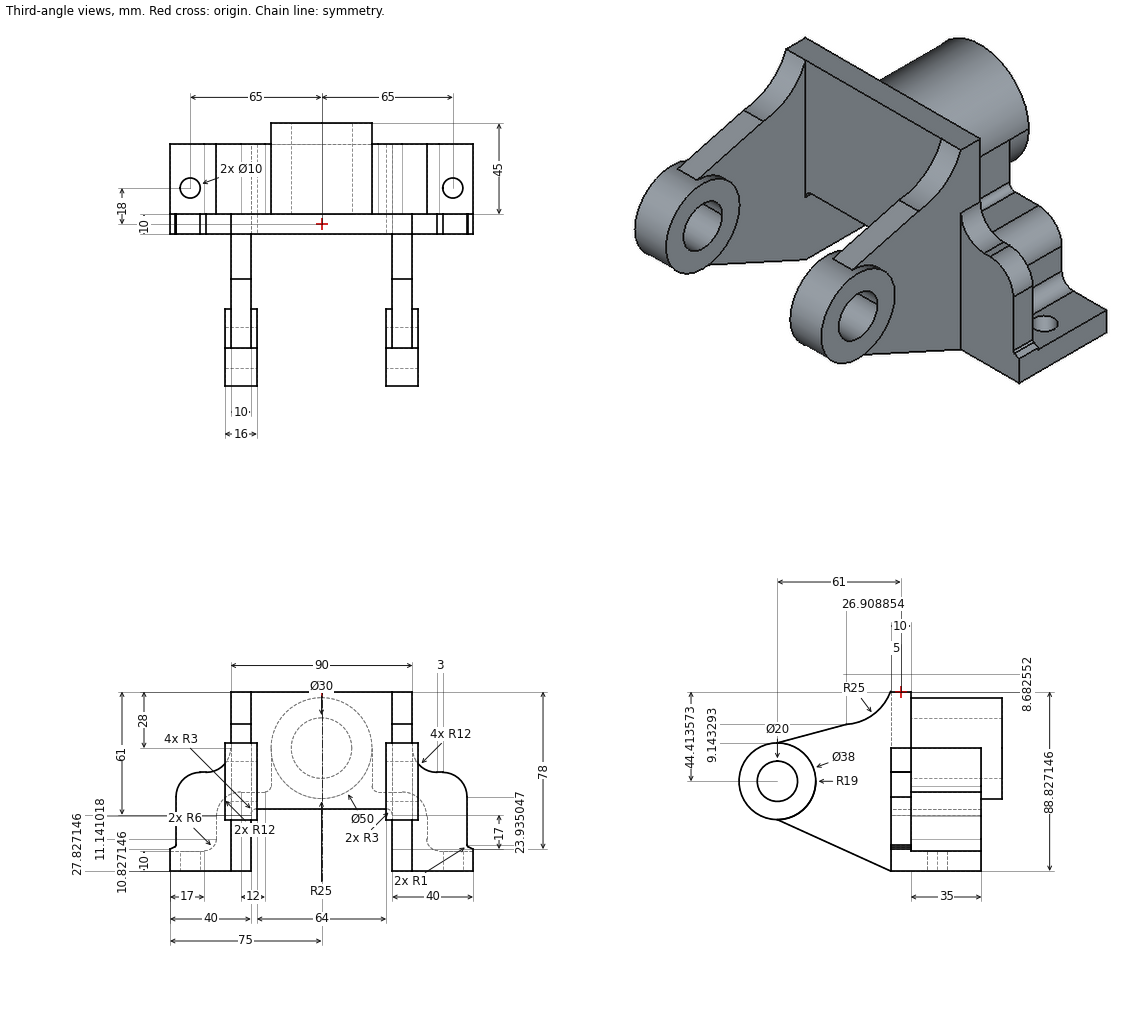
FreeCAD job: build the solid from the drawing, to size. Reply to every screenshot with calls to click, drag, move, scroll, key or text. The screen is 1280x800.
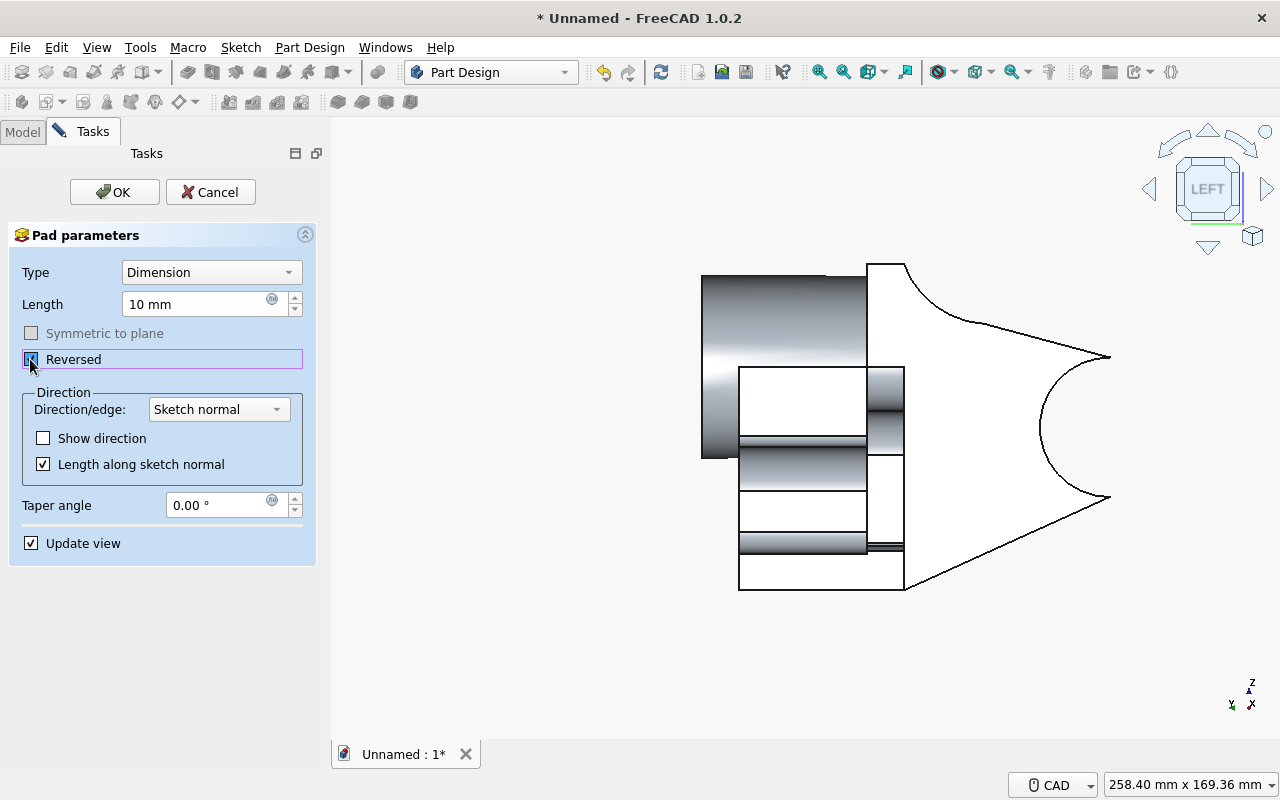
click(115, 192)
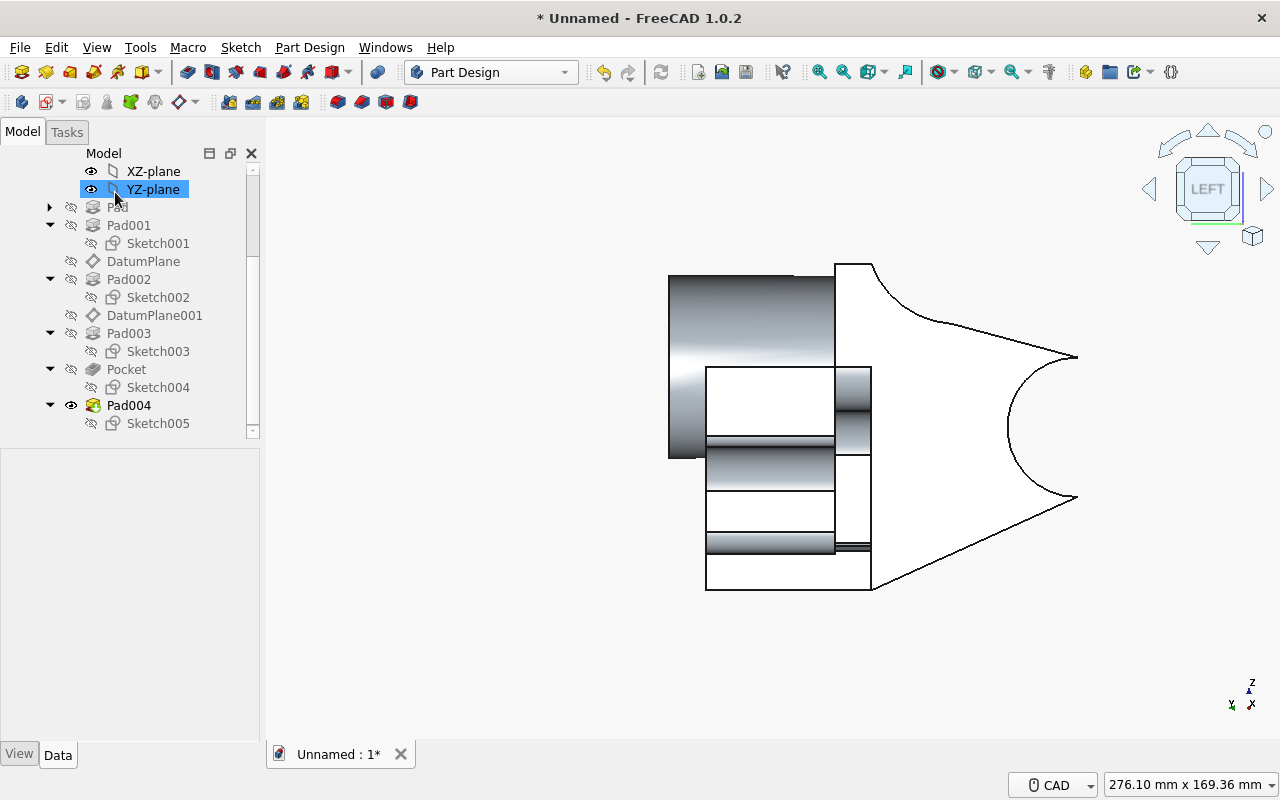
scroll(160, 293, down, 3)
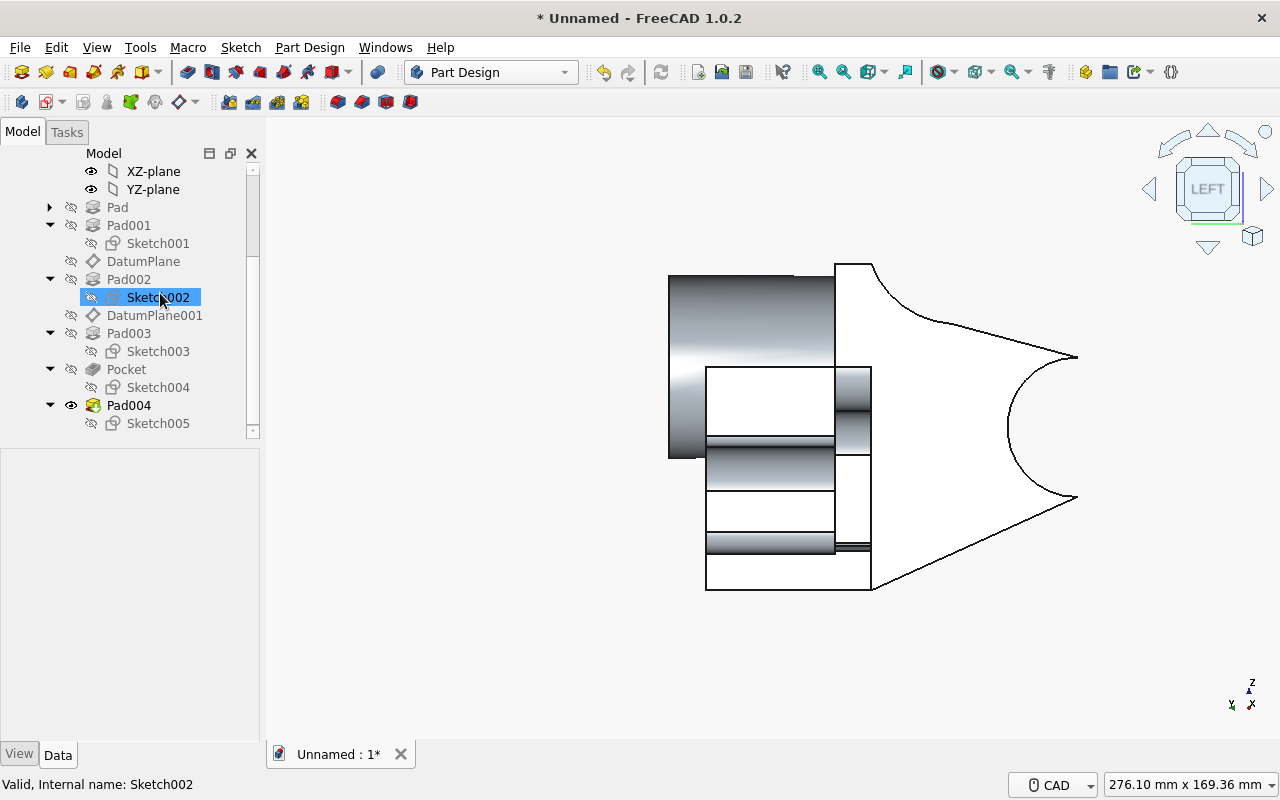
scroll(160, 293, up, 15)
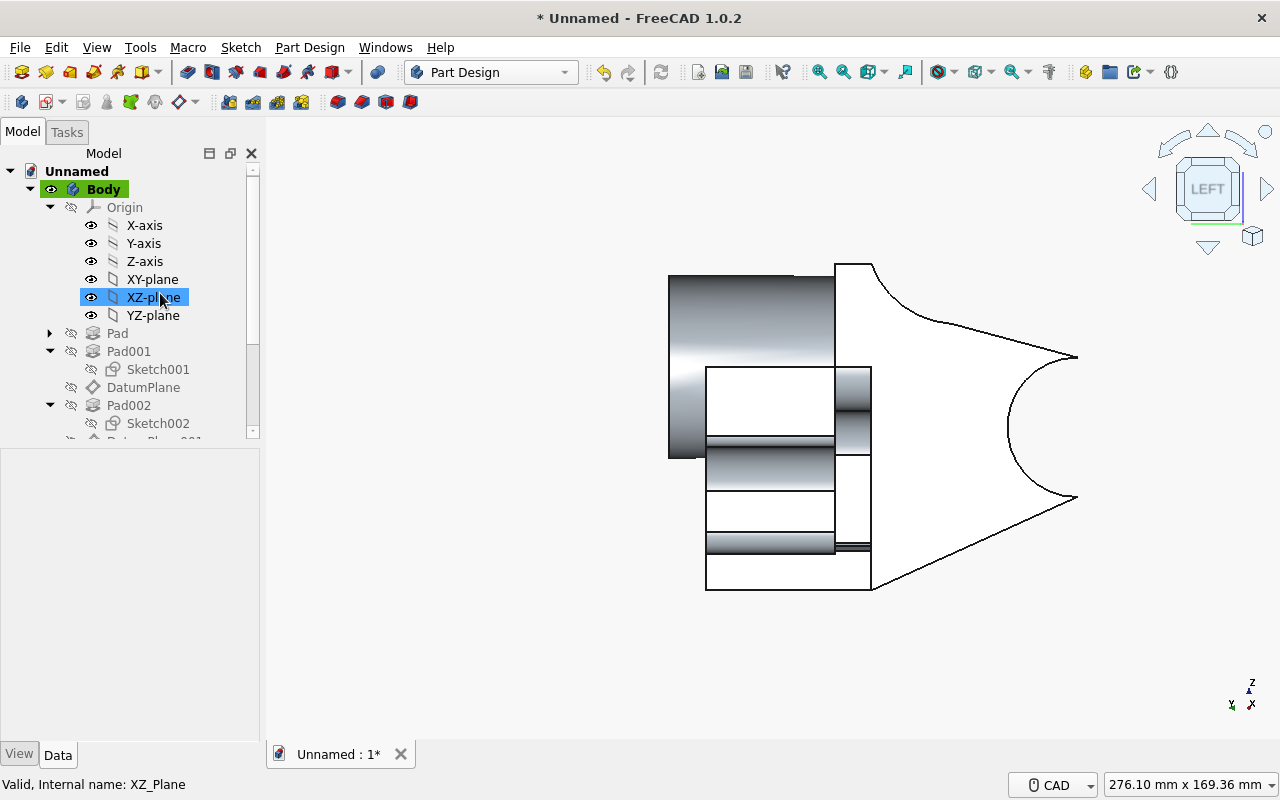
click(136, 315)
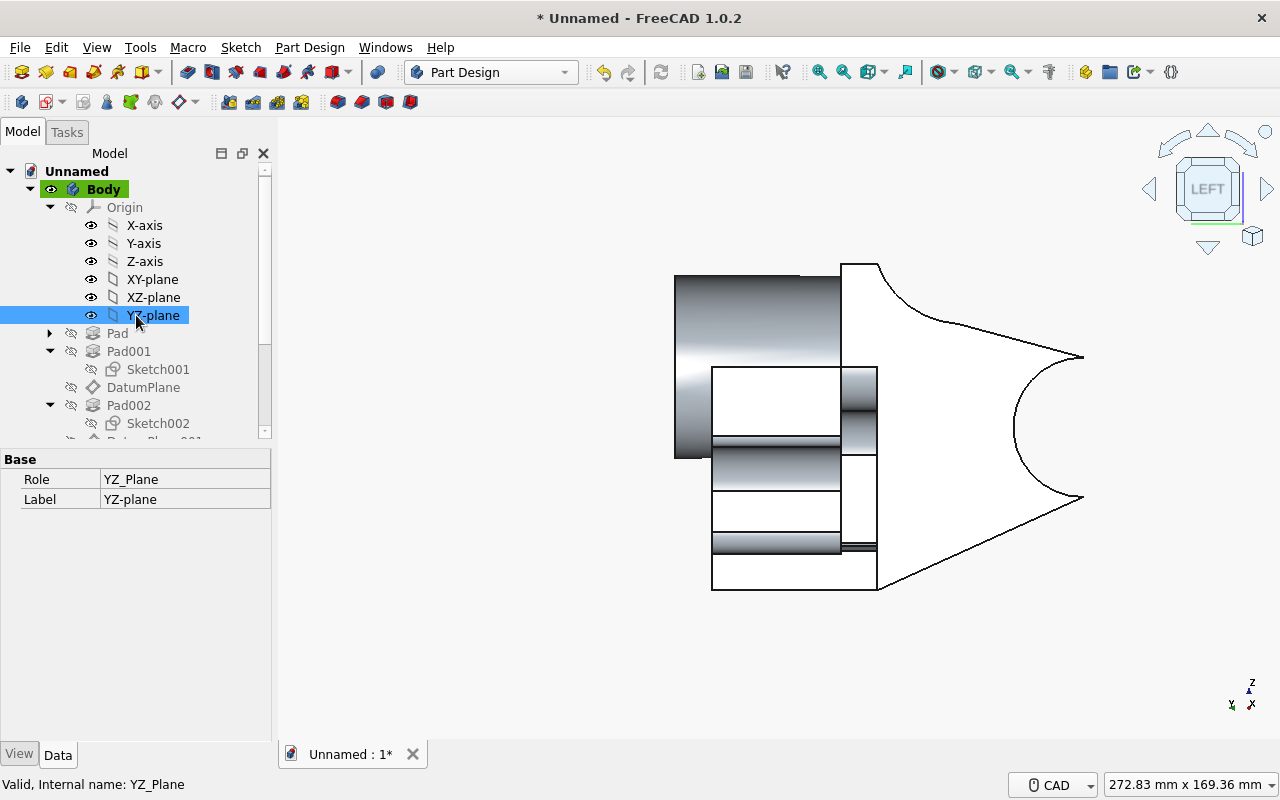
click(180, 102)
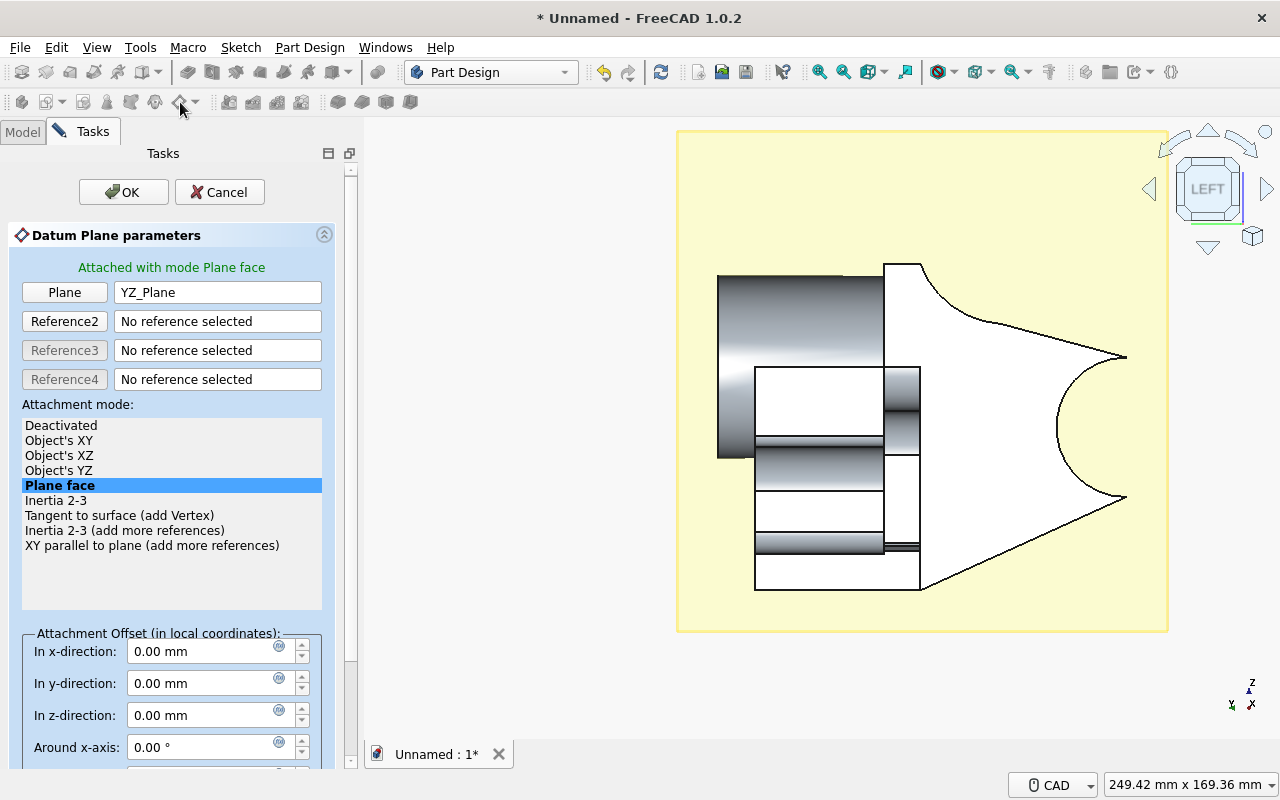
triple_click(210, 715)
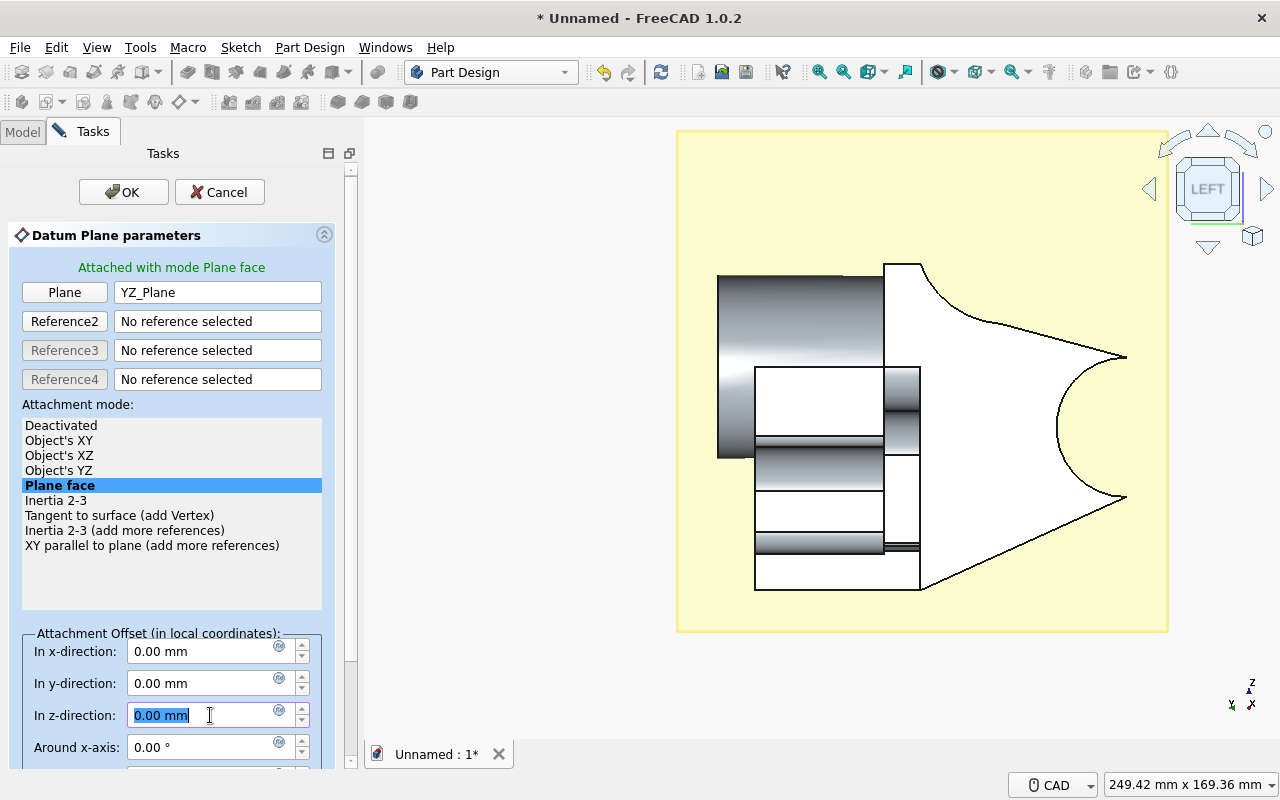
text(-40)
key(Tab)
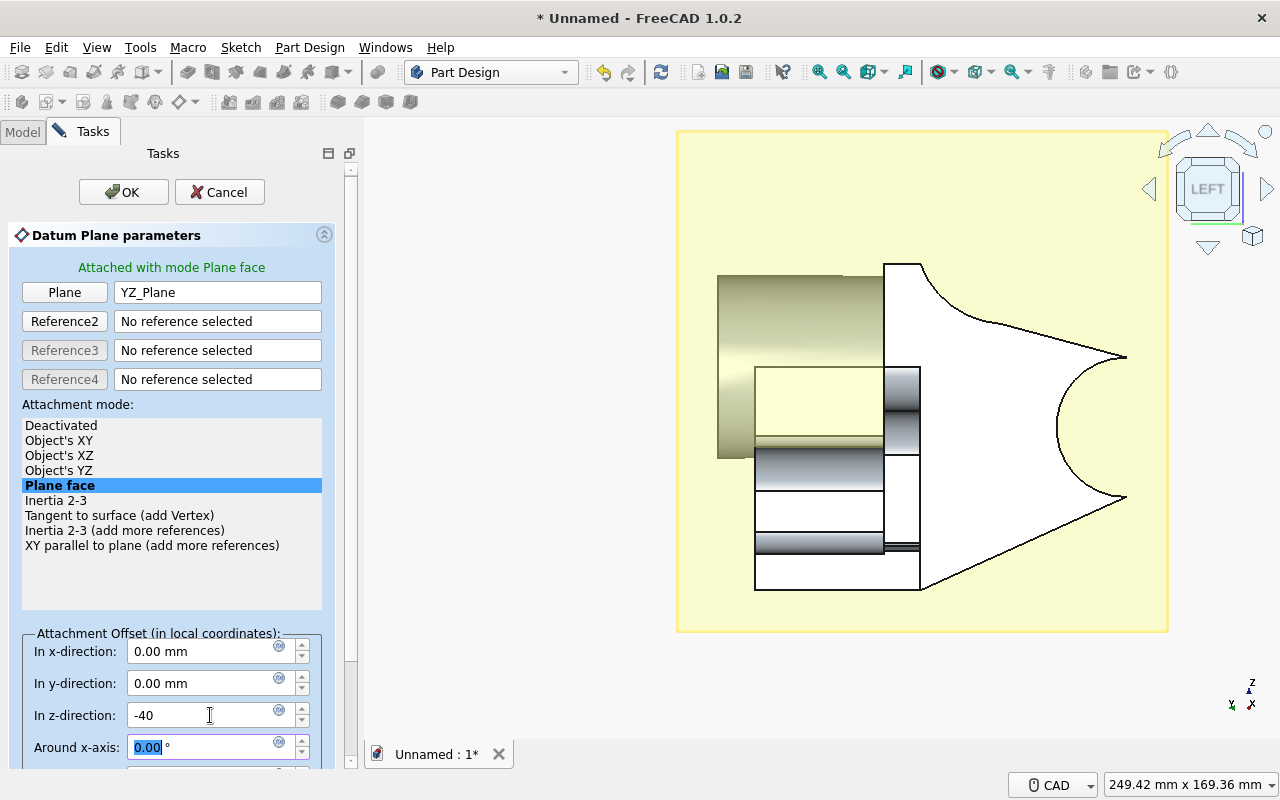
click(124, 192)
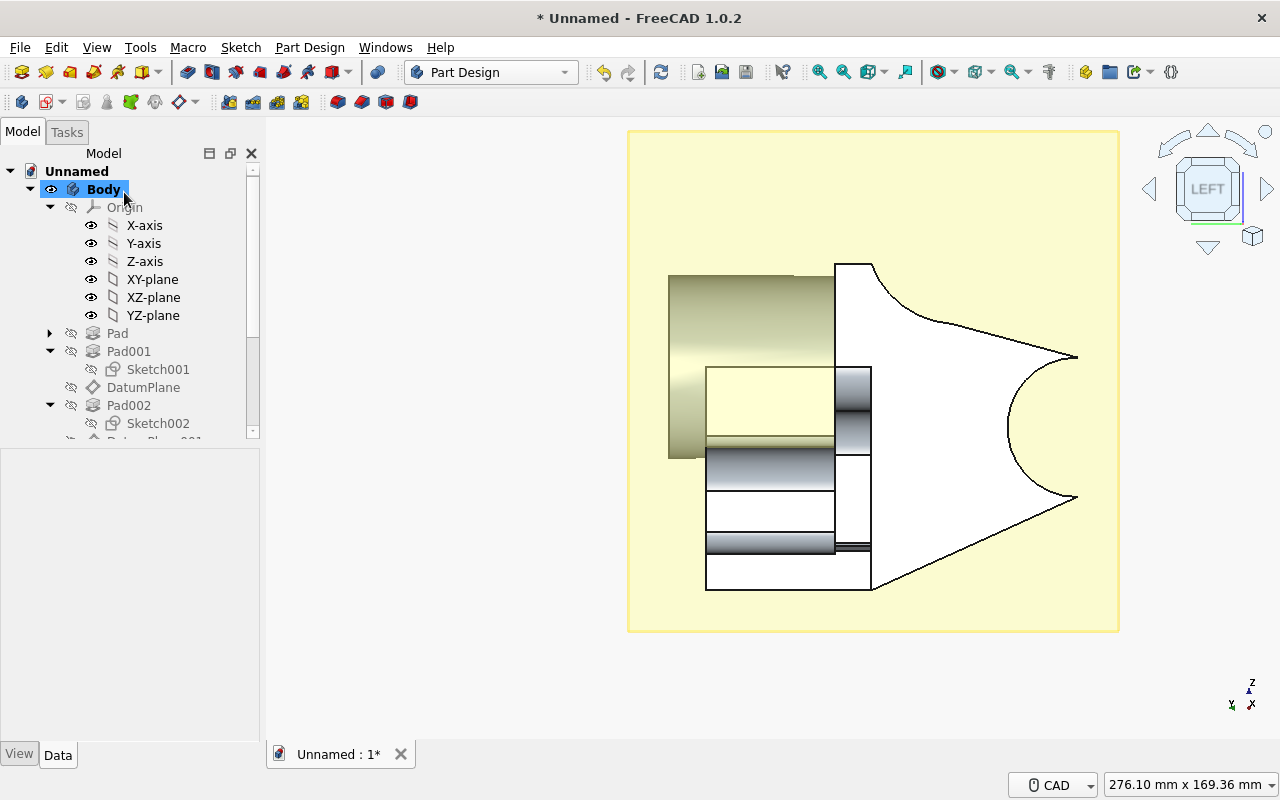
scroll(100, 293, down, 3)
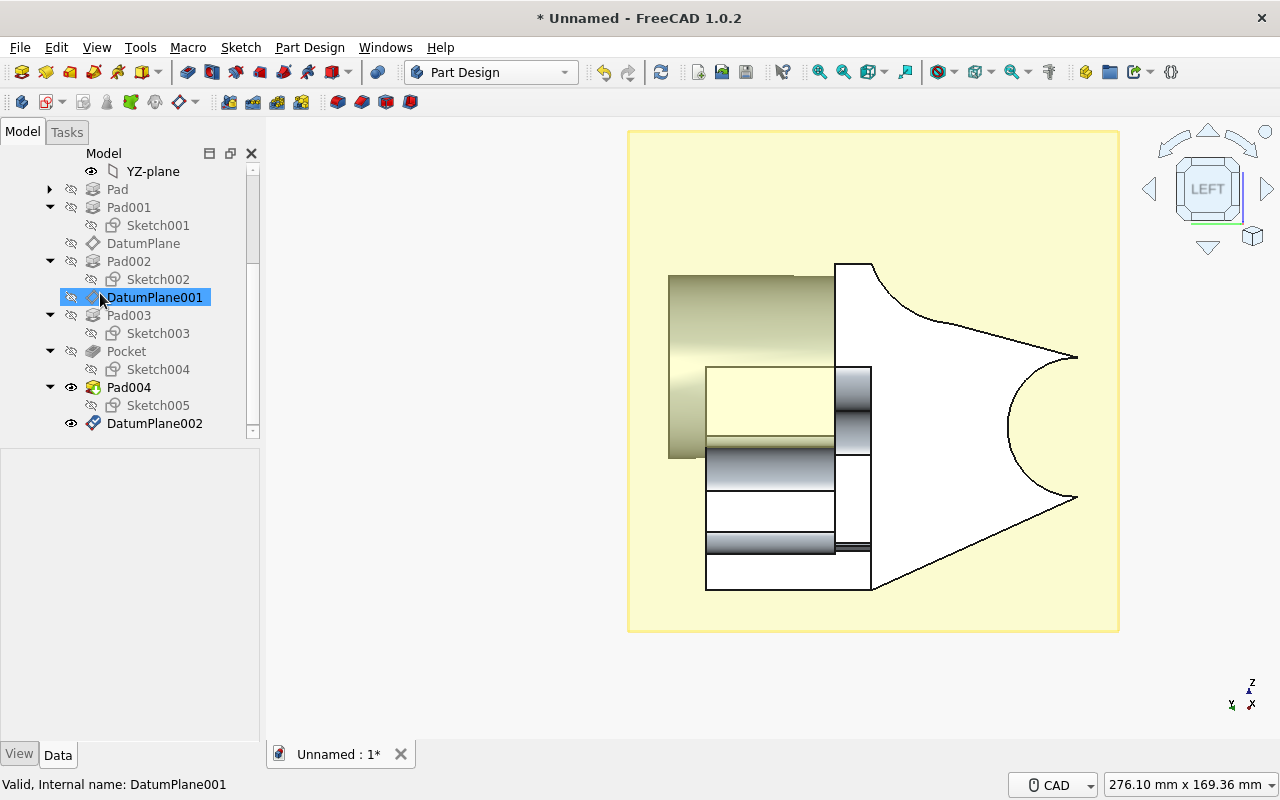
click(116, 423)